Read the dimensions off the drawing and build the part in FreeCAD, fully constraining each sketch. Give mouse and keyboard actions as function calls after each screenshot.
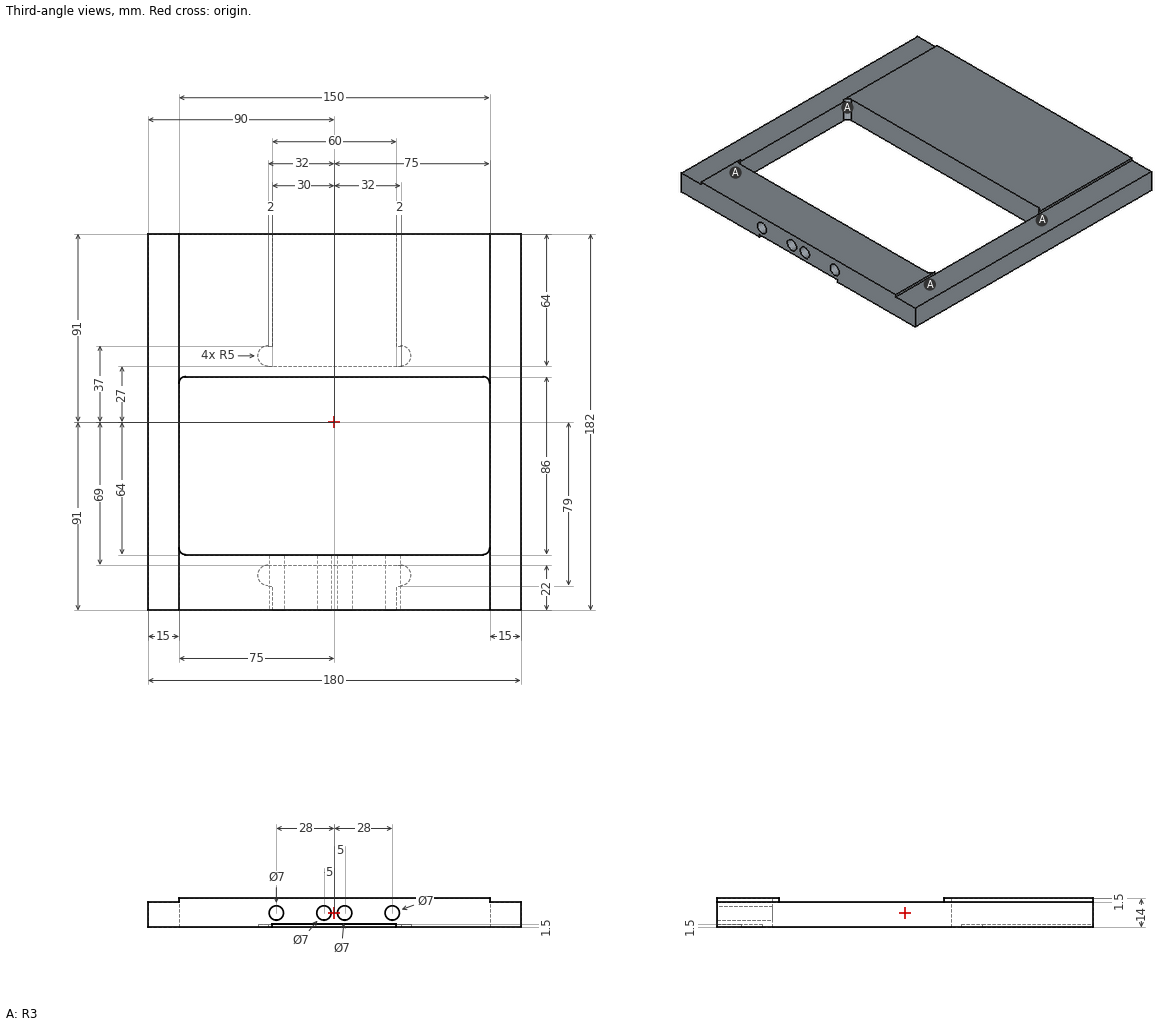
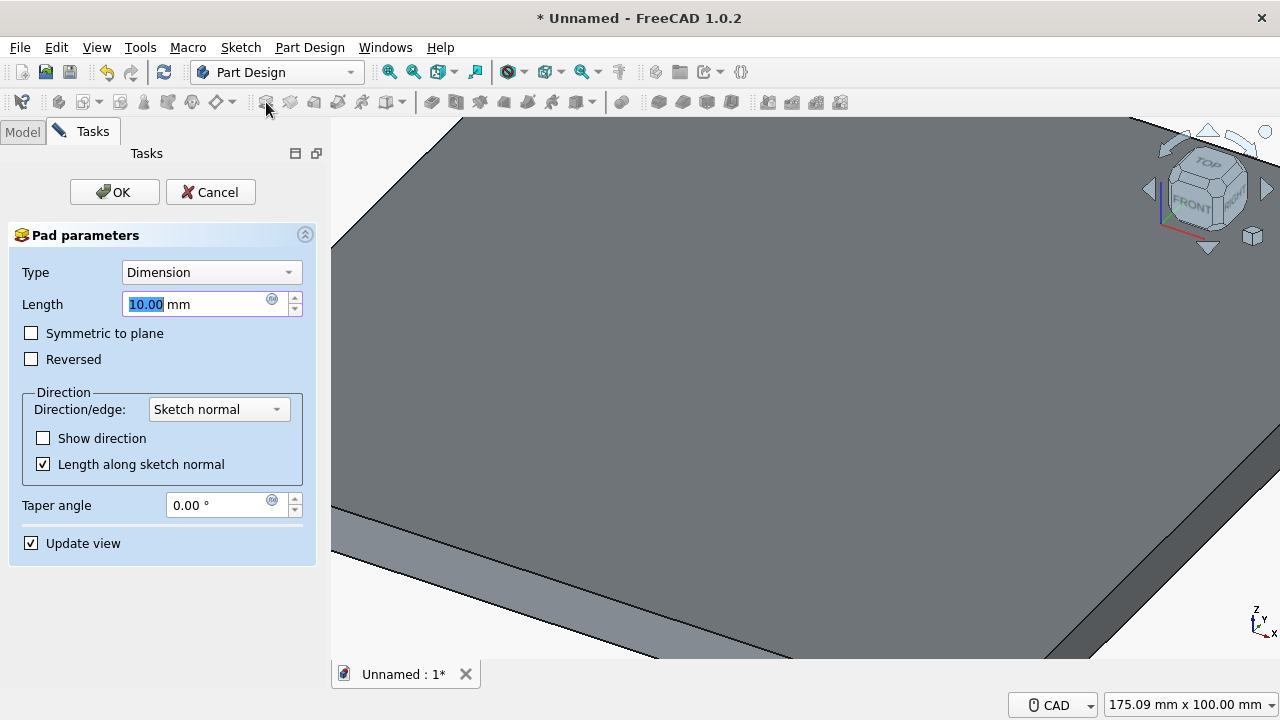
text(14)
key(Tab)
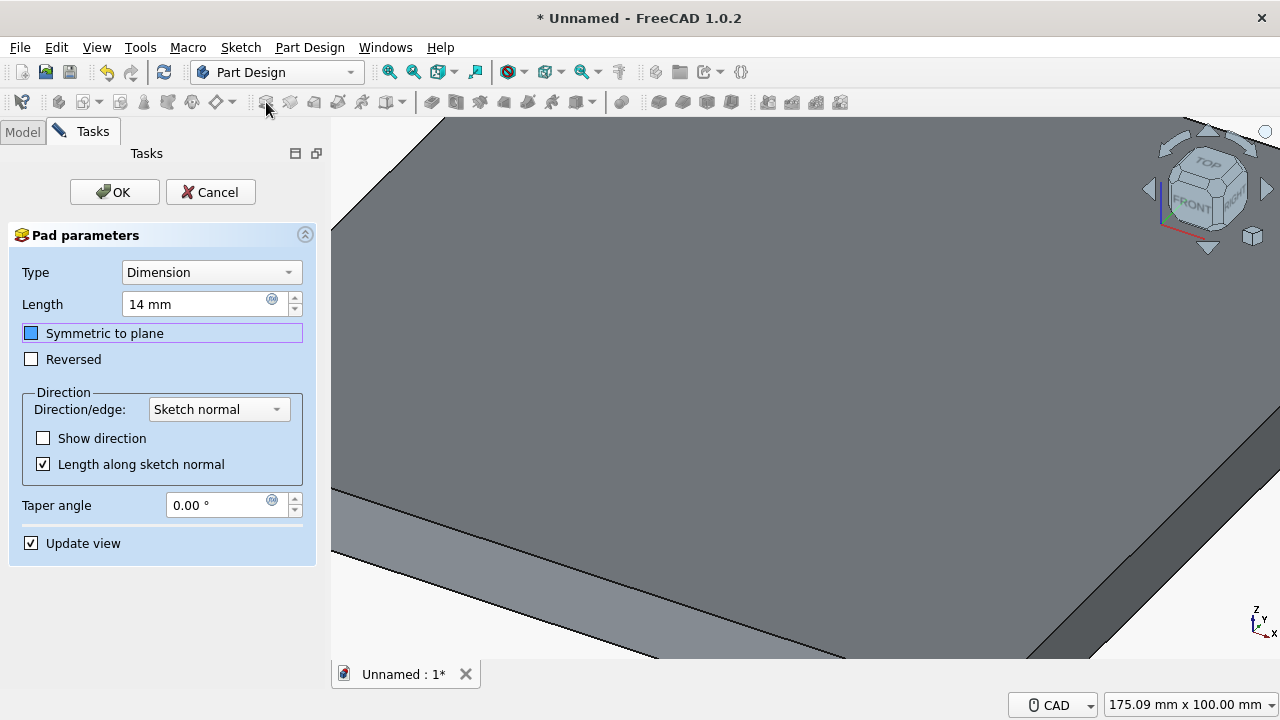
click(30, 333)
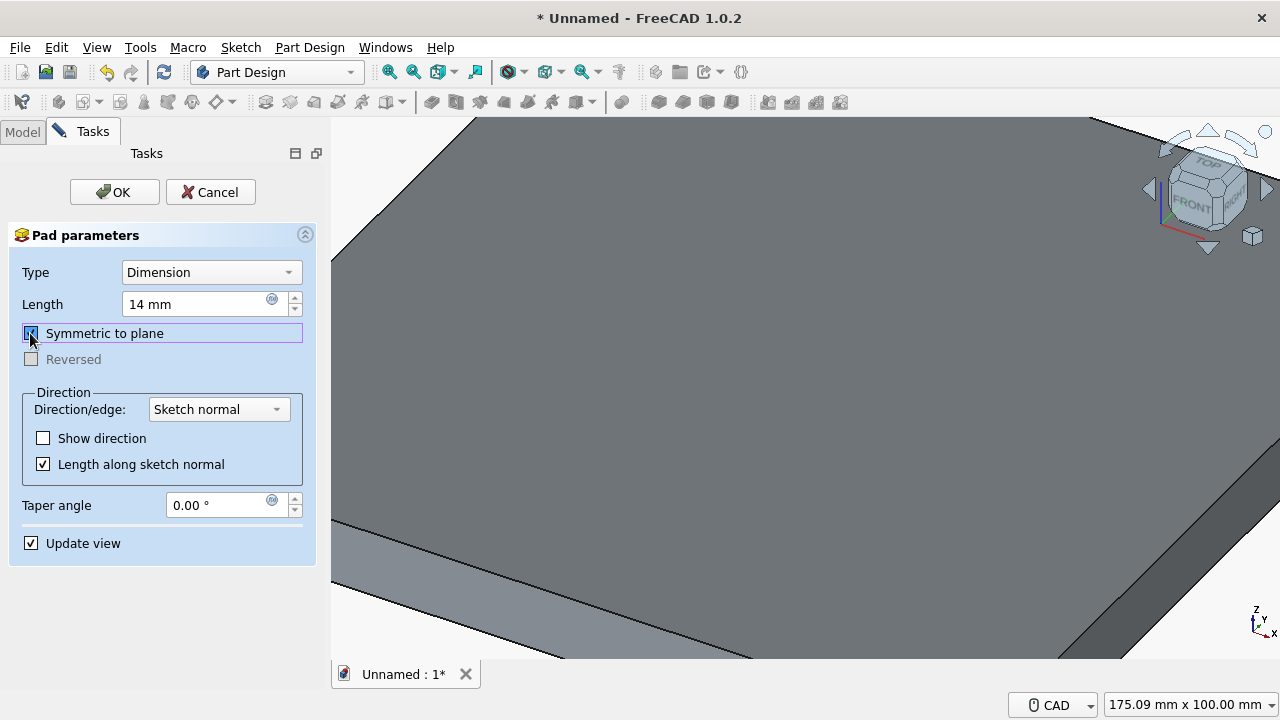
click(115, 192)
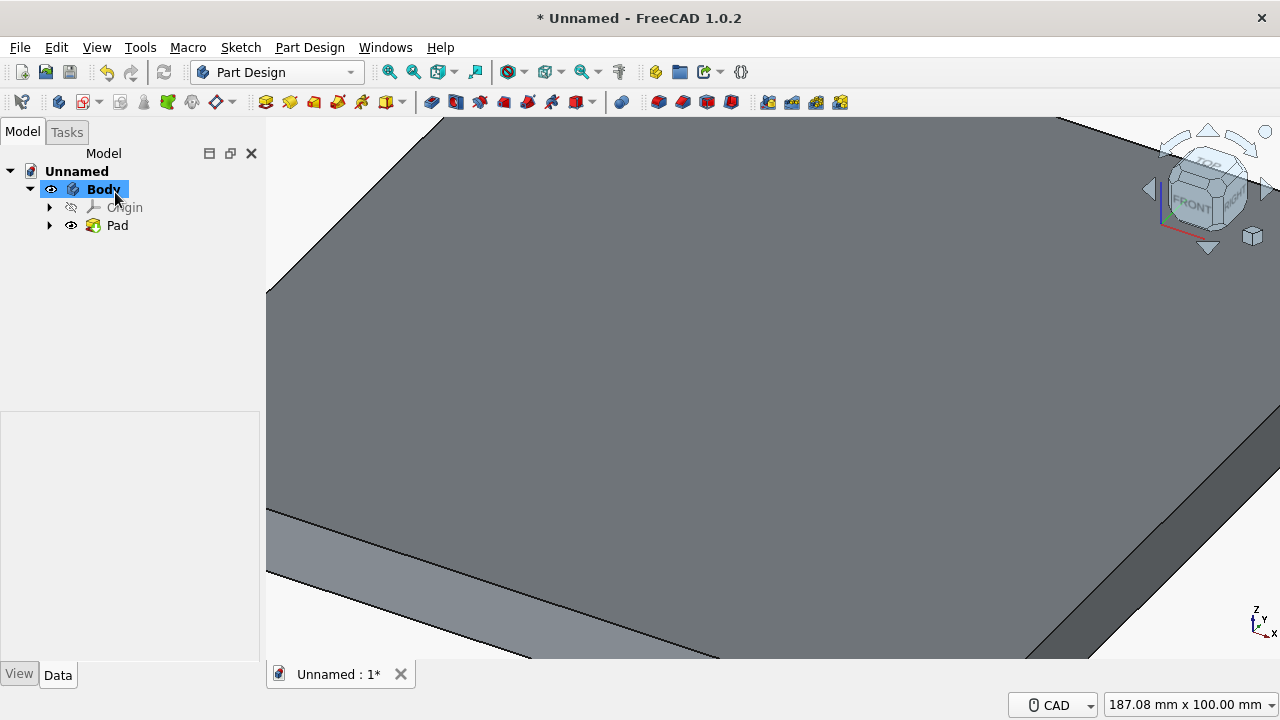
click(390, 72)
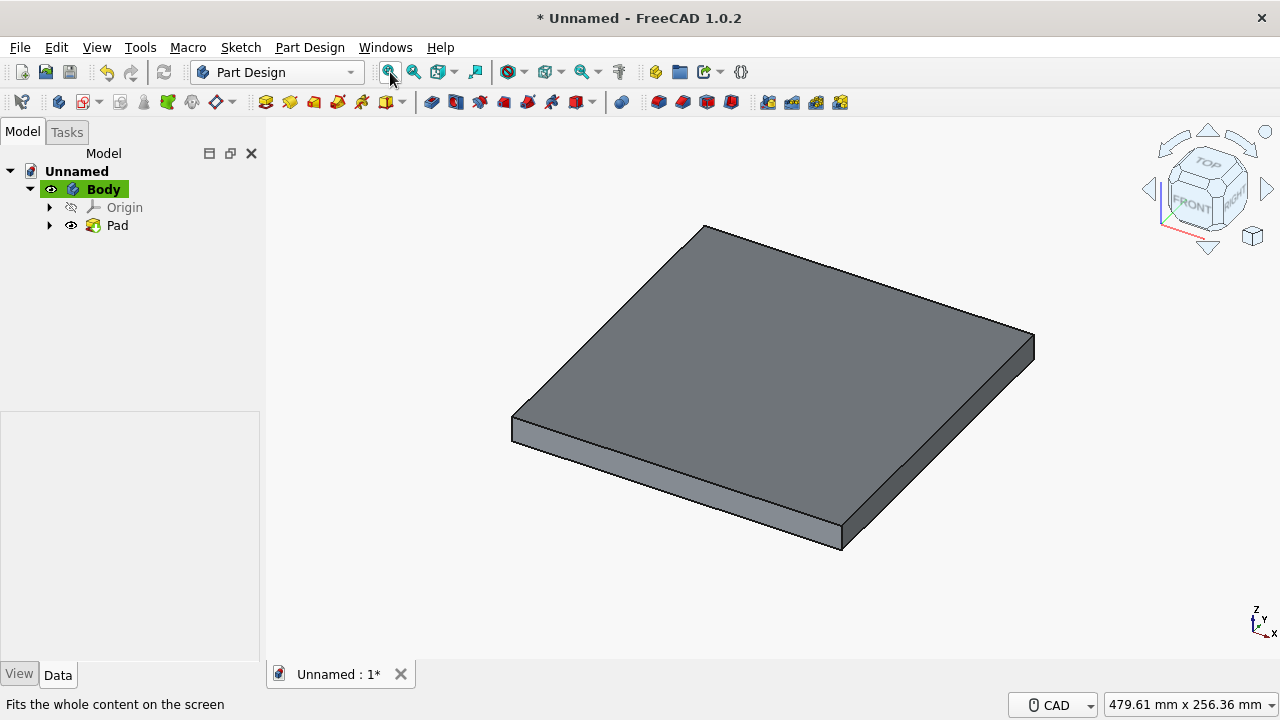
key(5)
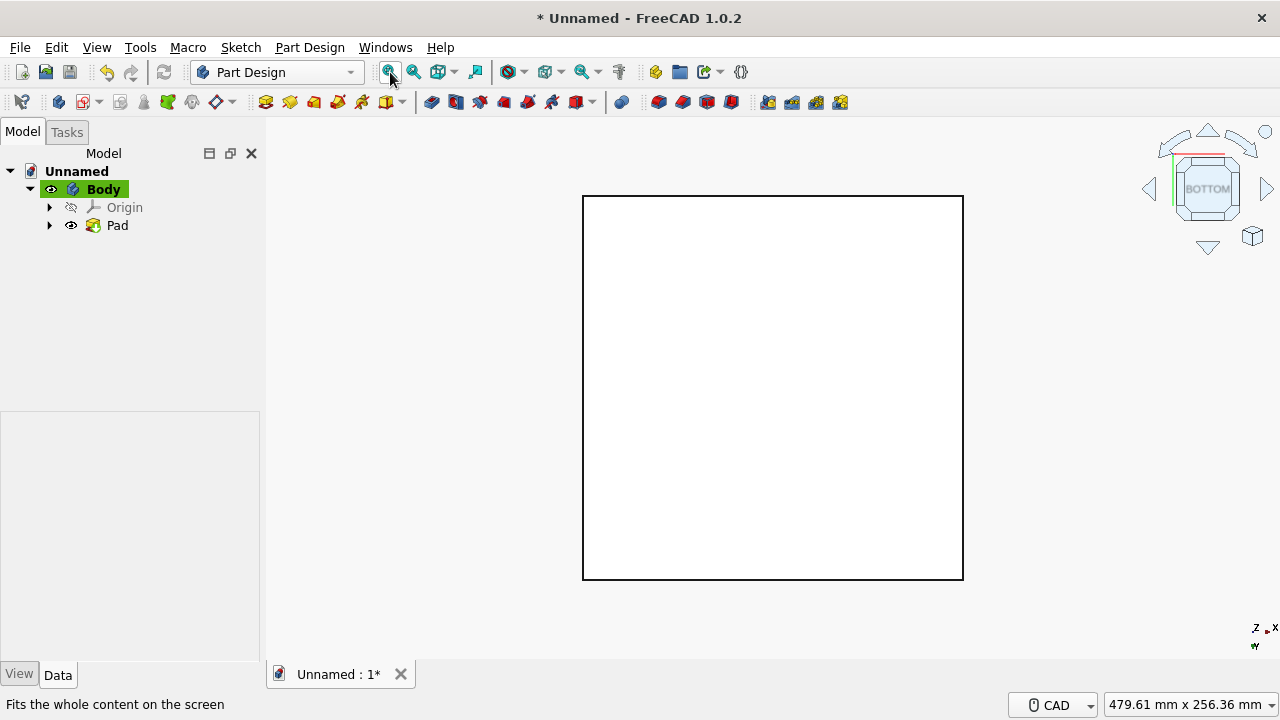
click(773, 387)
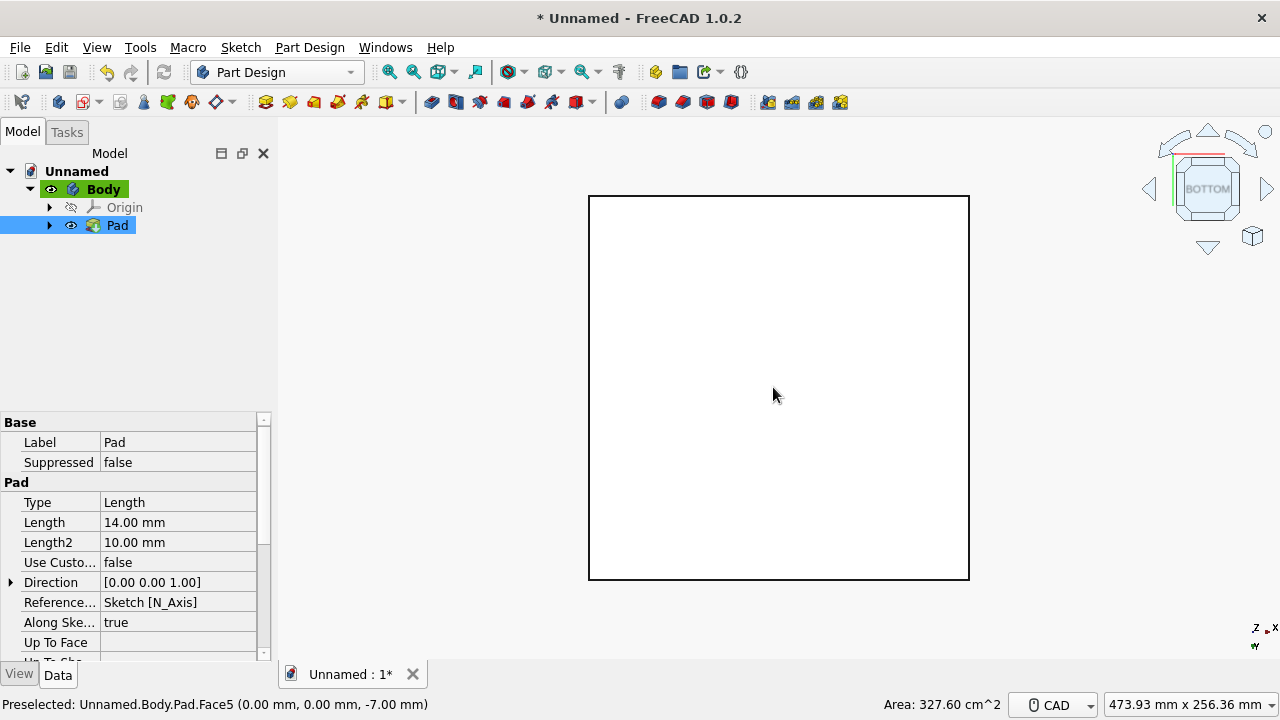
click(84, 102)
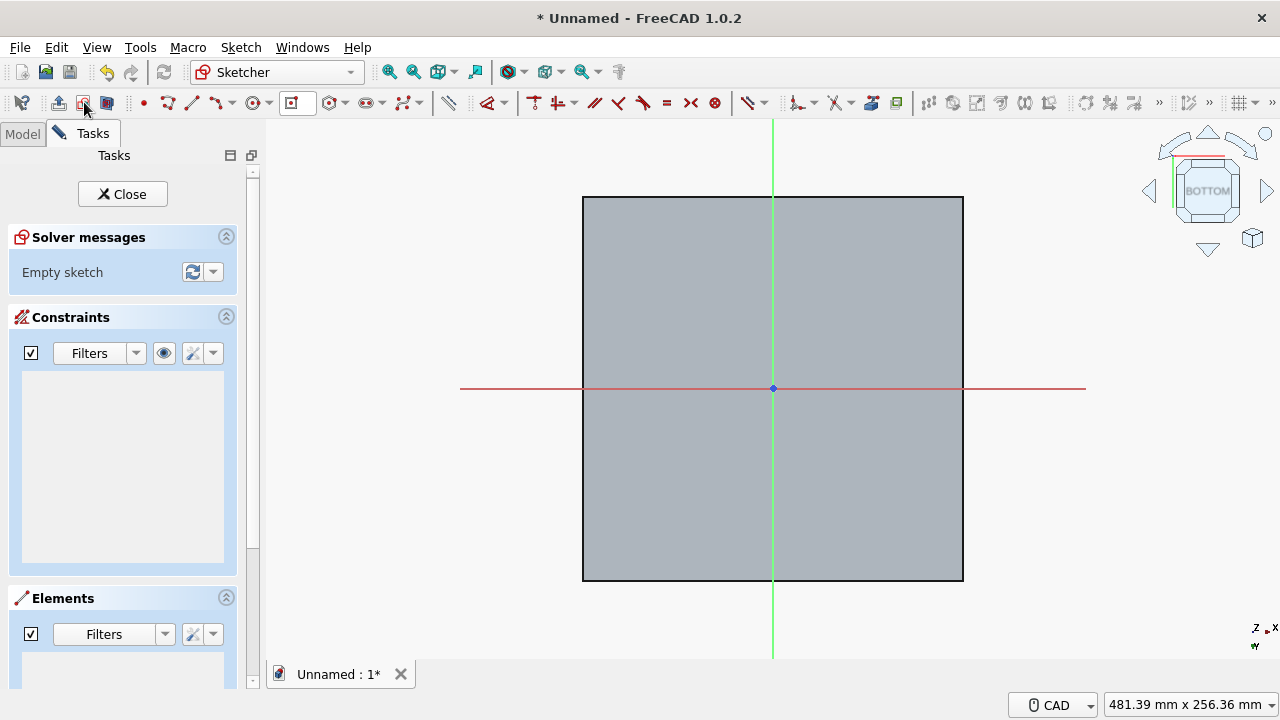
key(g)
key(r)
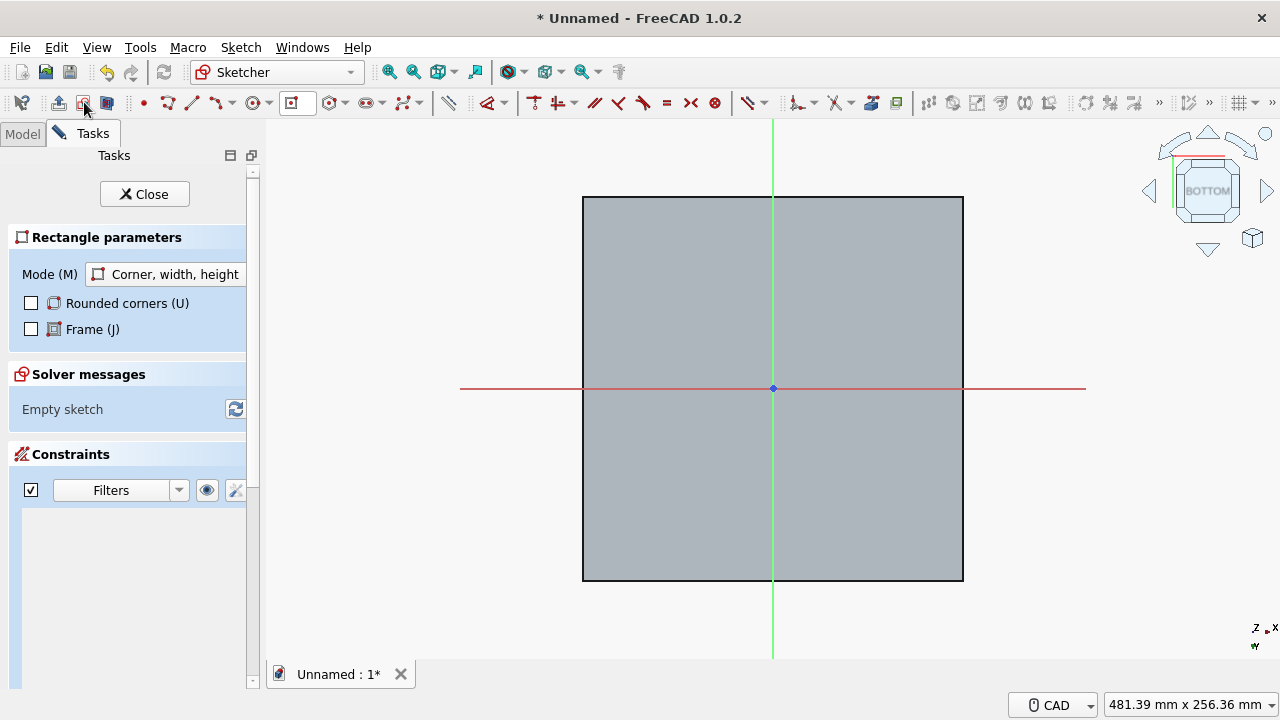
click(710, 446)
move(836, 581)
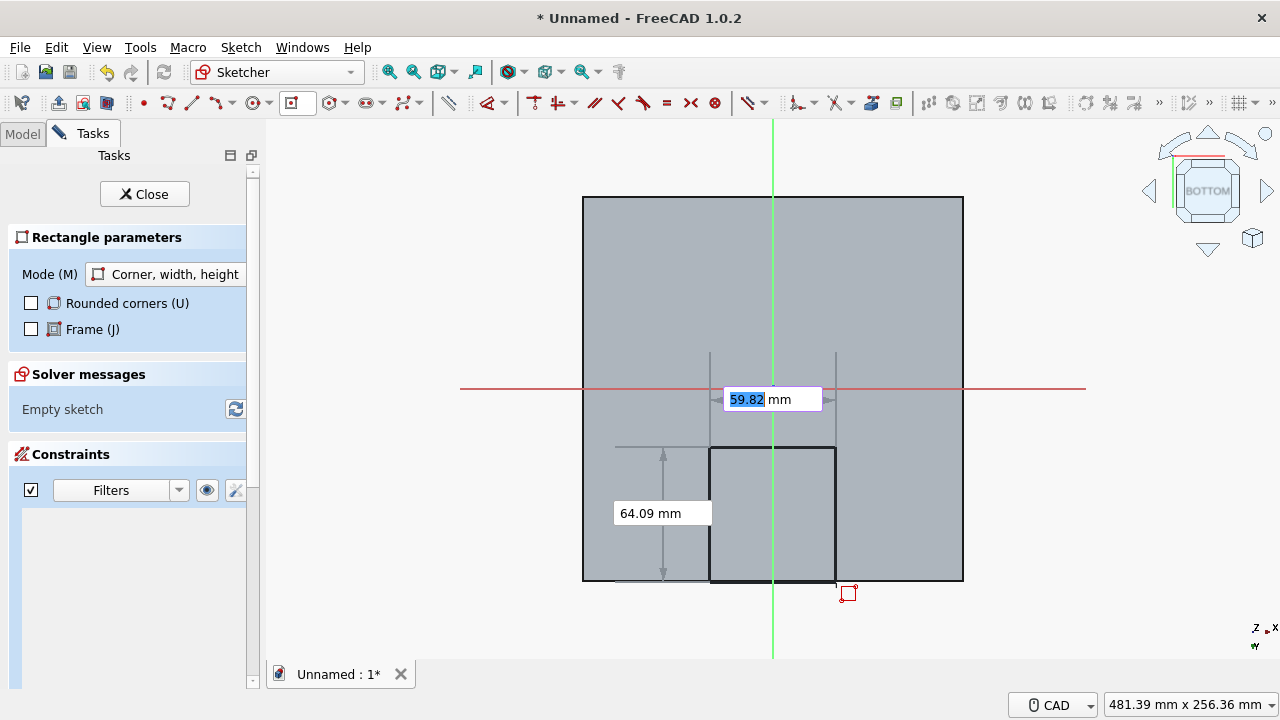
text(60)
key(Tab)
text(64)
key(Return)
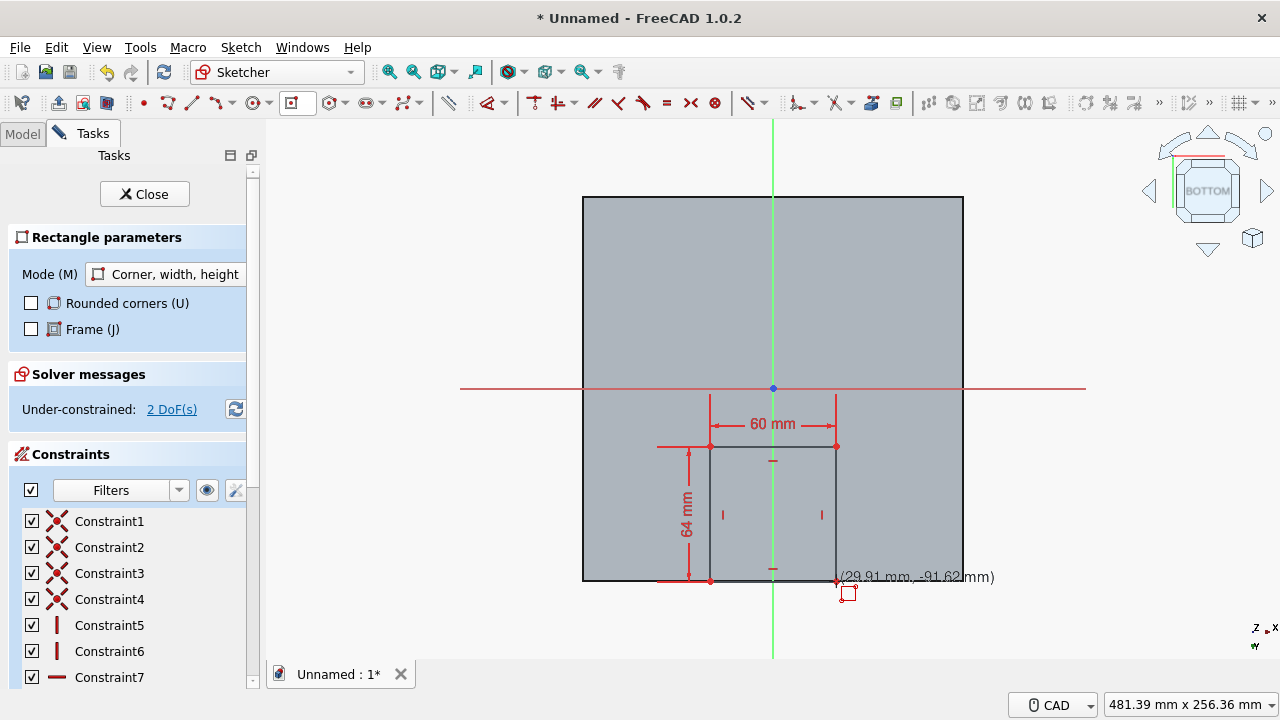
click(710, 197)
move(836, 244)